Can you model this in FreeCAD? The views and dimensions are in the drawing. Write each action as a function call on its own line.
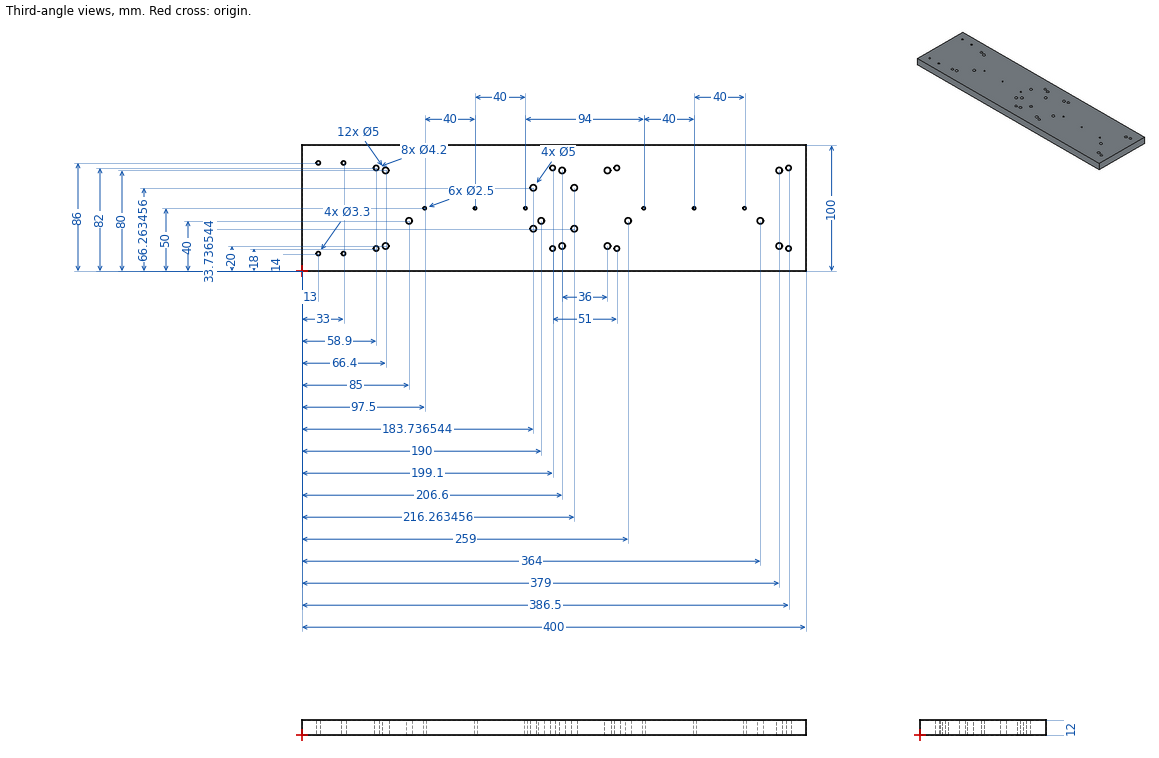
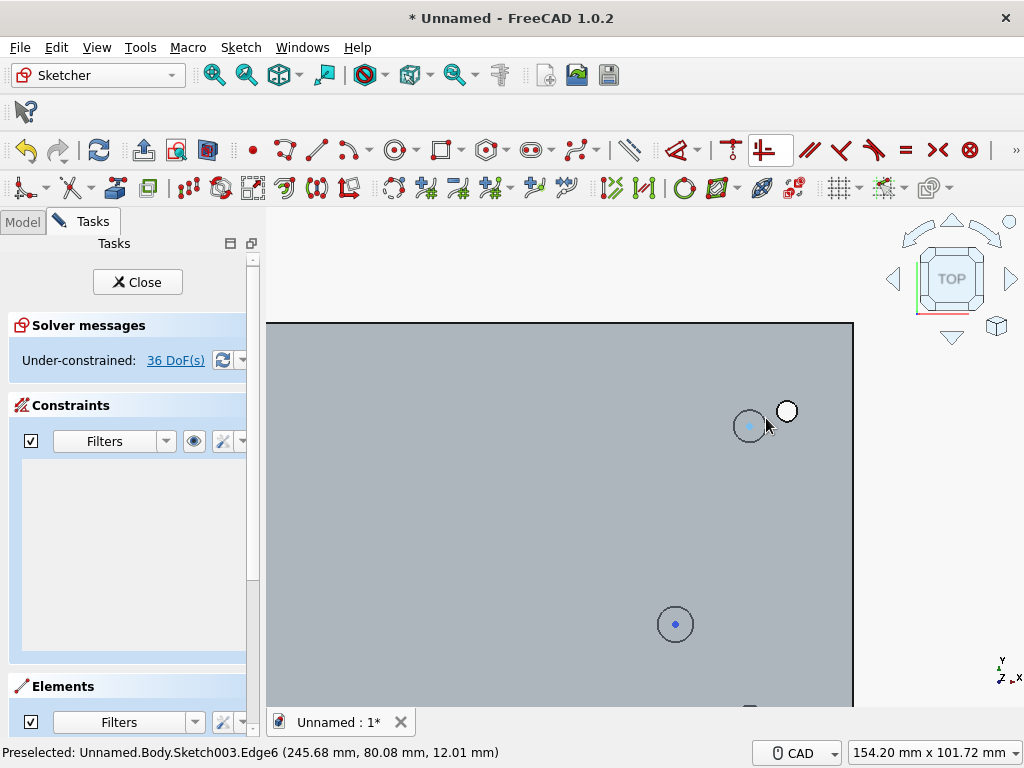
click(761, 415)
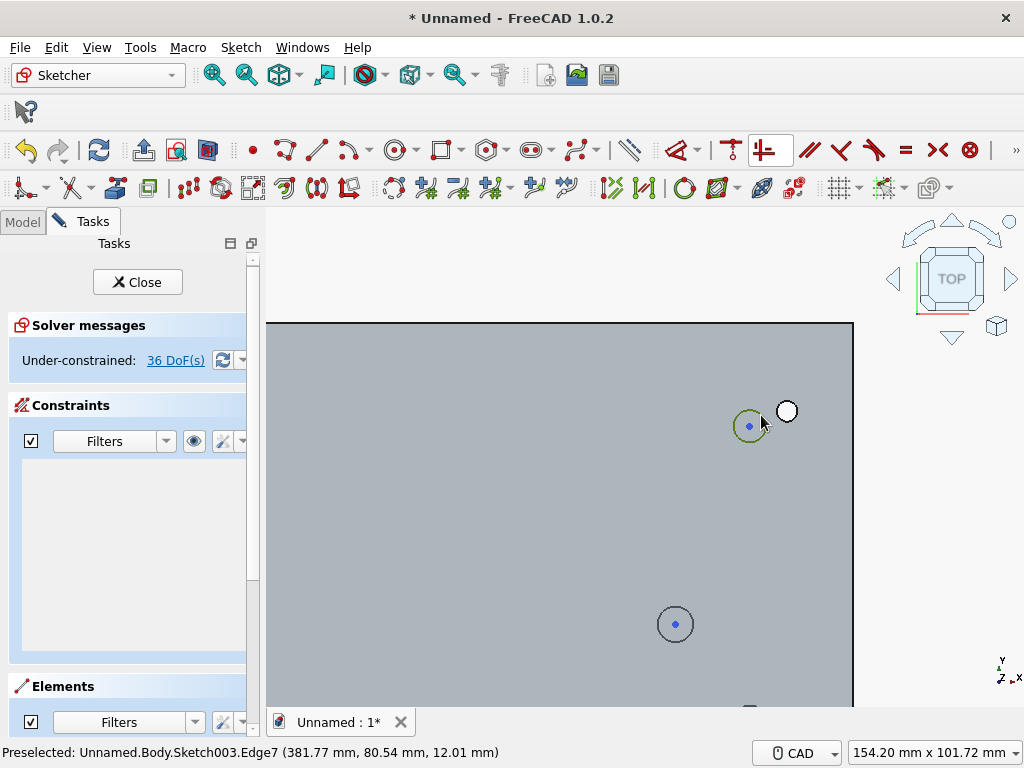
scroll(767, 418, down, 8)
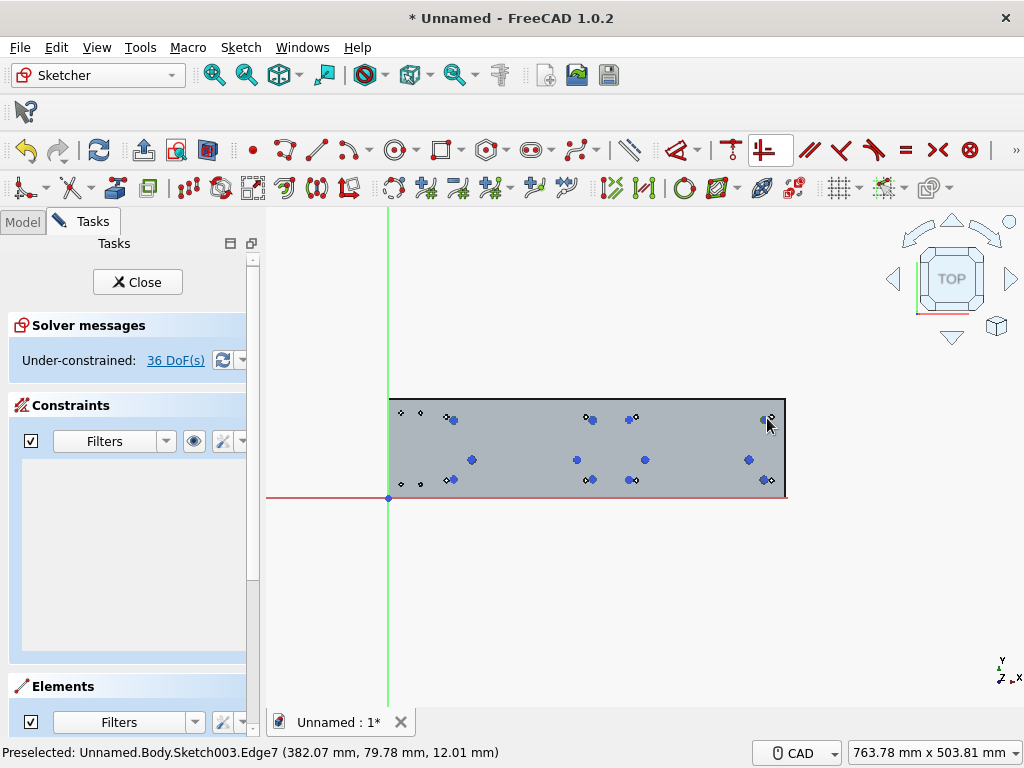
scroll(767, 477, up, 7)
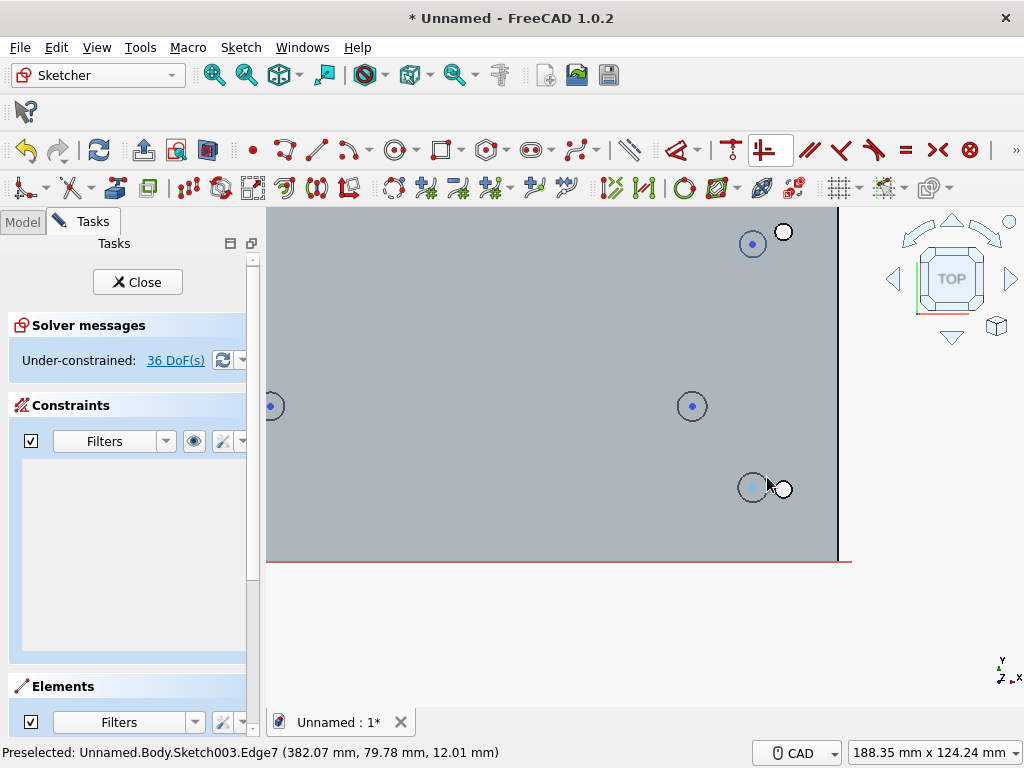
click(763, 477)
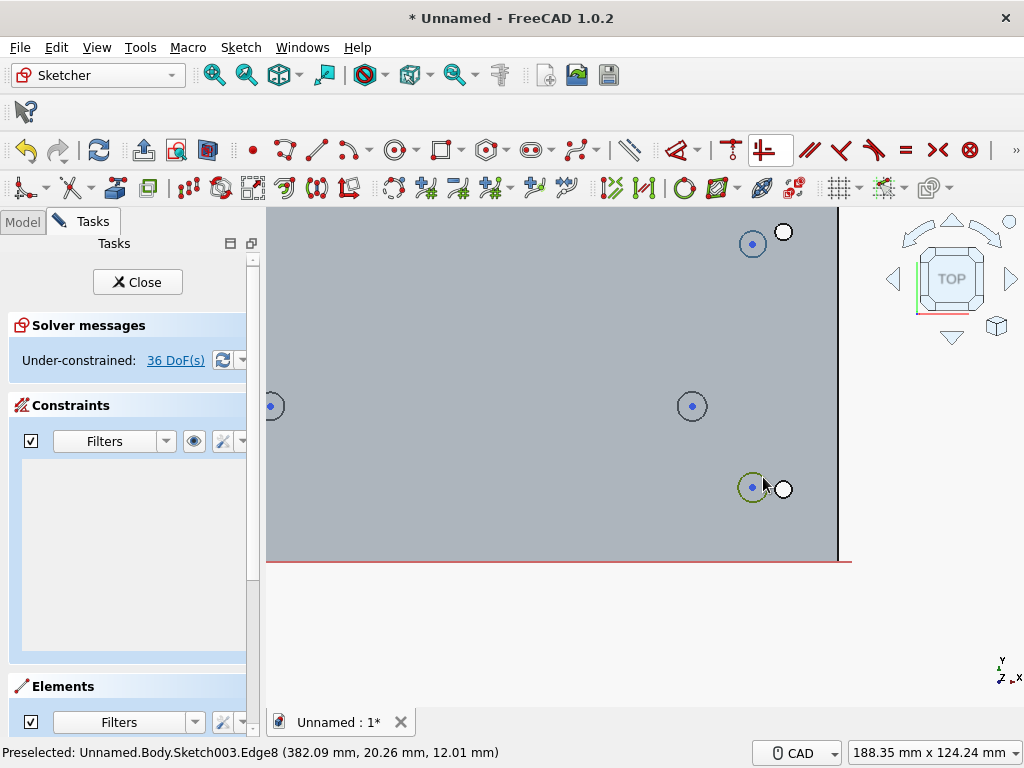
scroll(767, 477, down, 7)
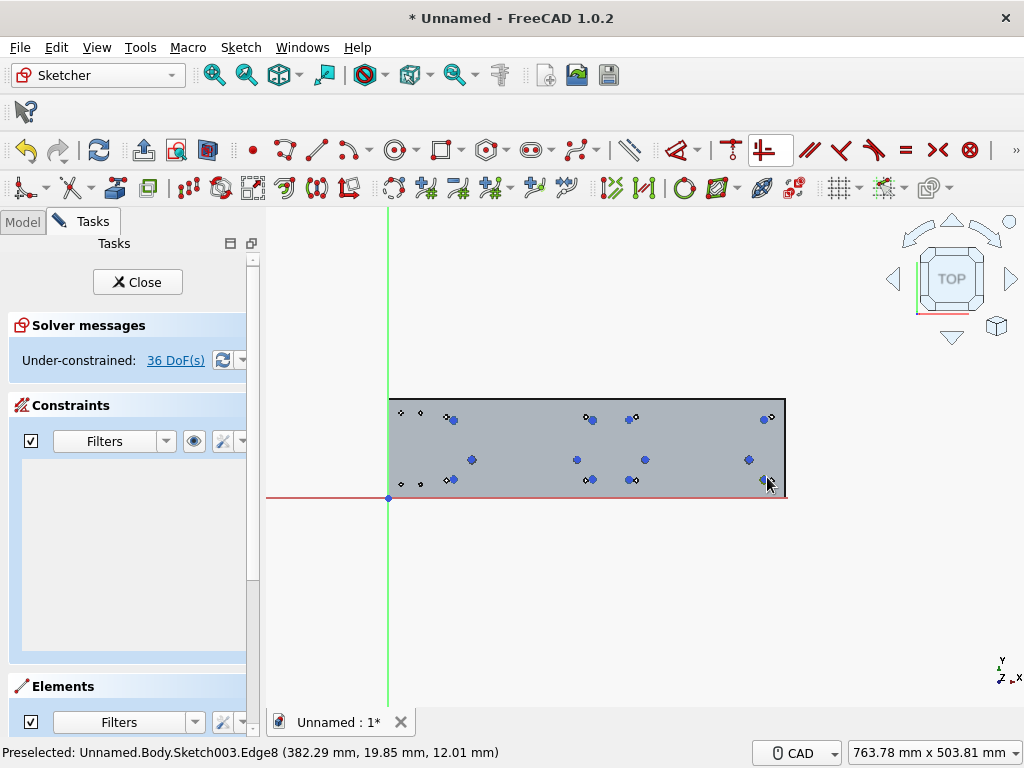
scroll(475, 457, up, 7)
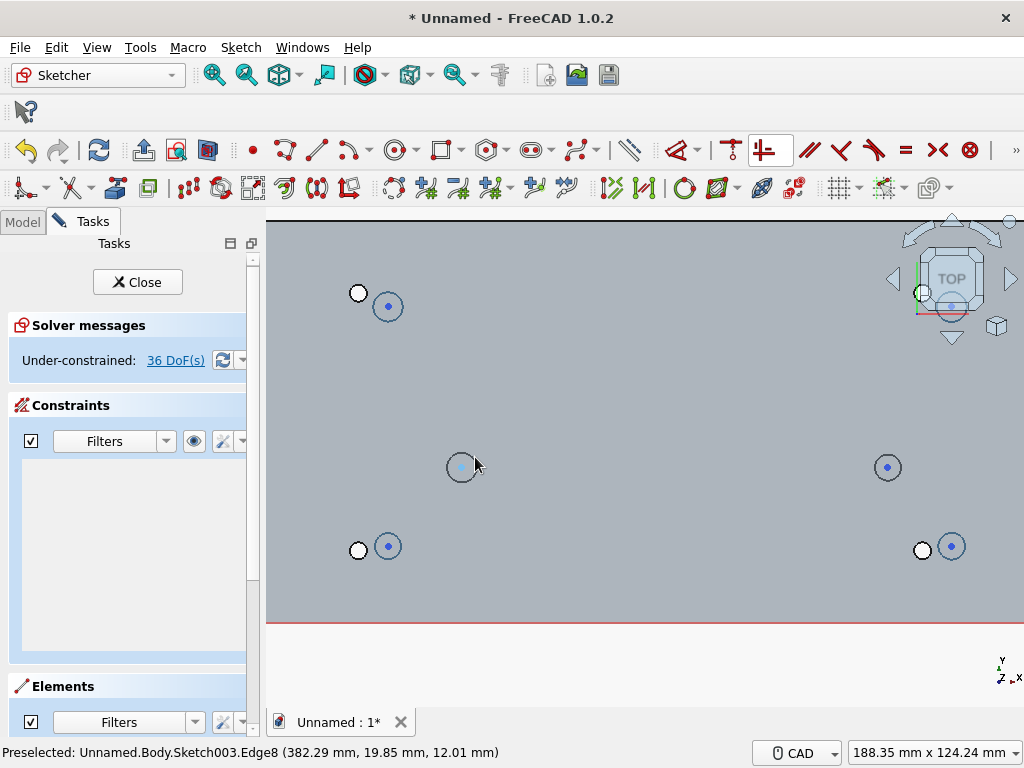
click(472, 457)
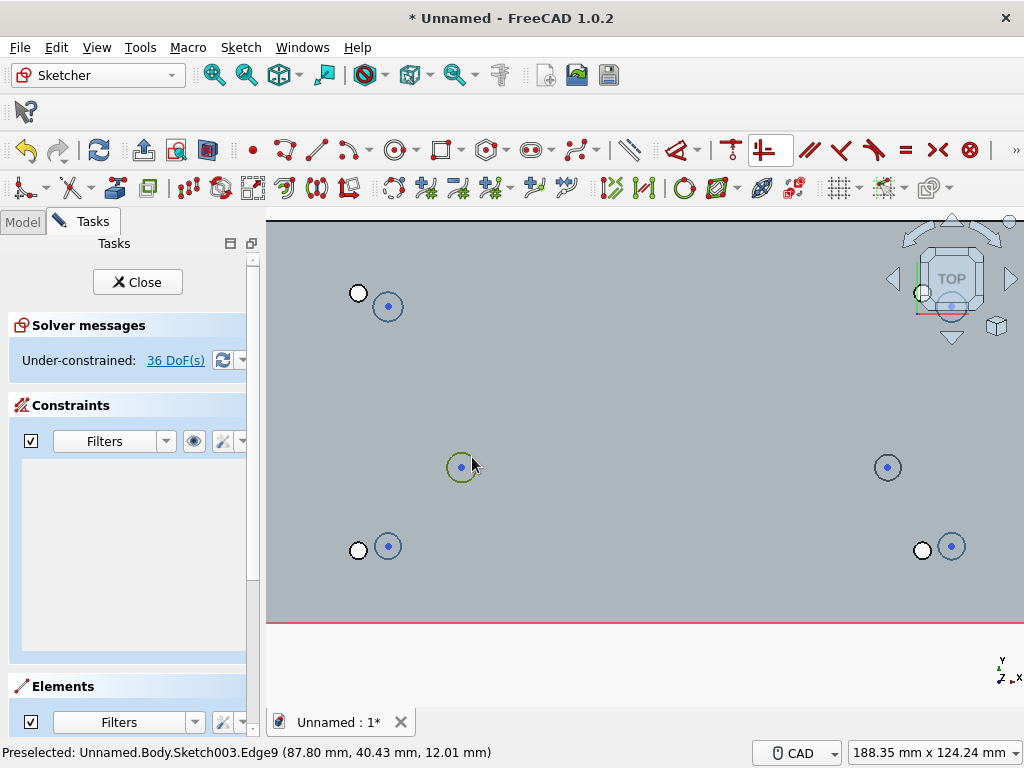
scroll(474, 457, down, 7)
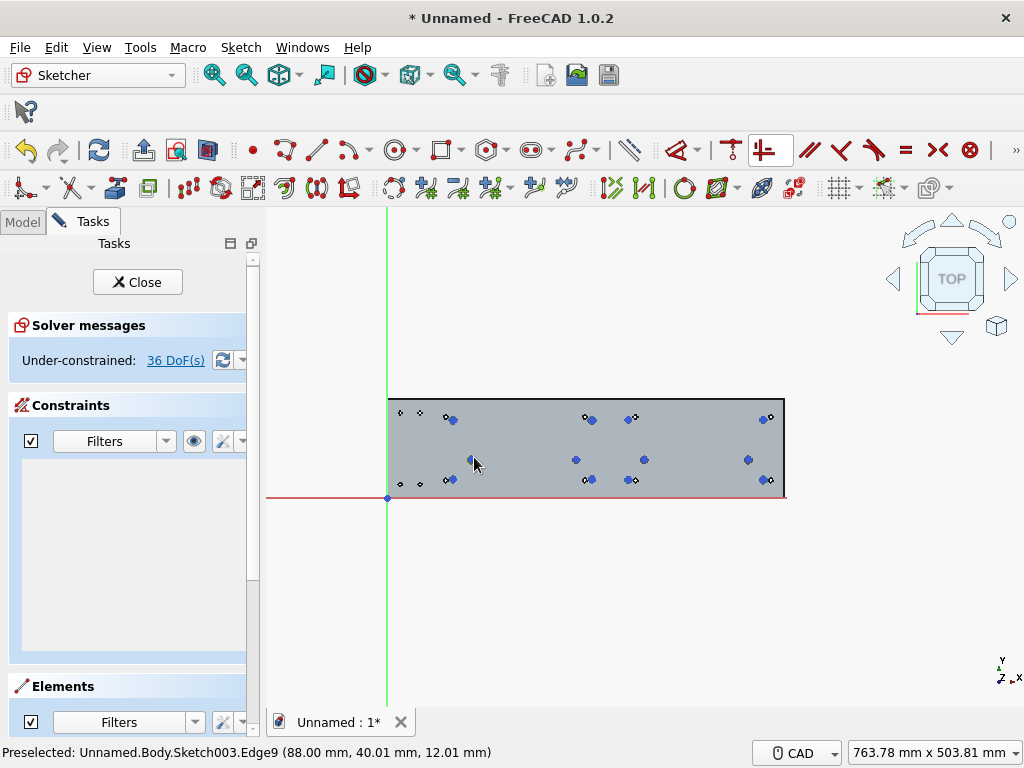
scroll(579, 458, up, 8)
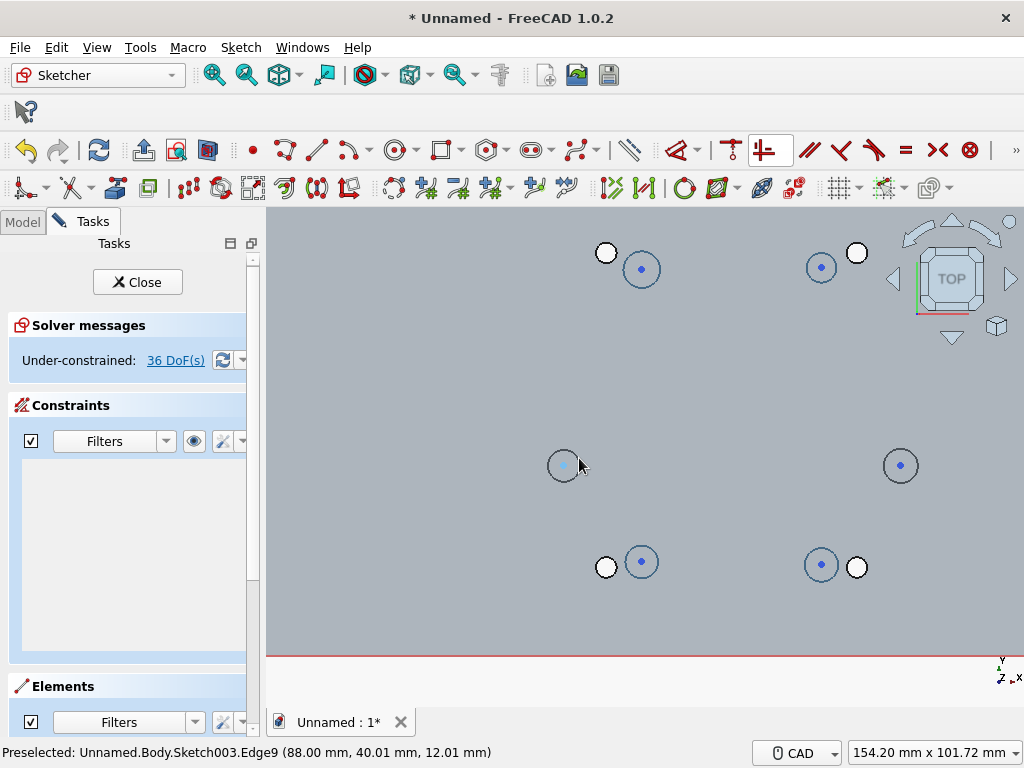
click(575, 455)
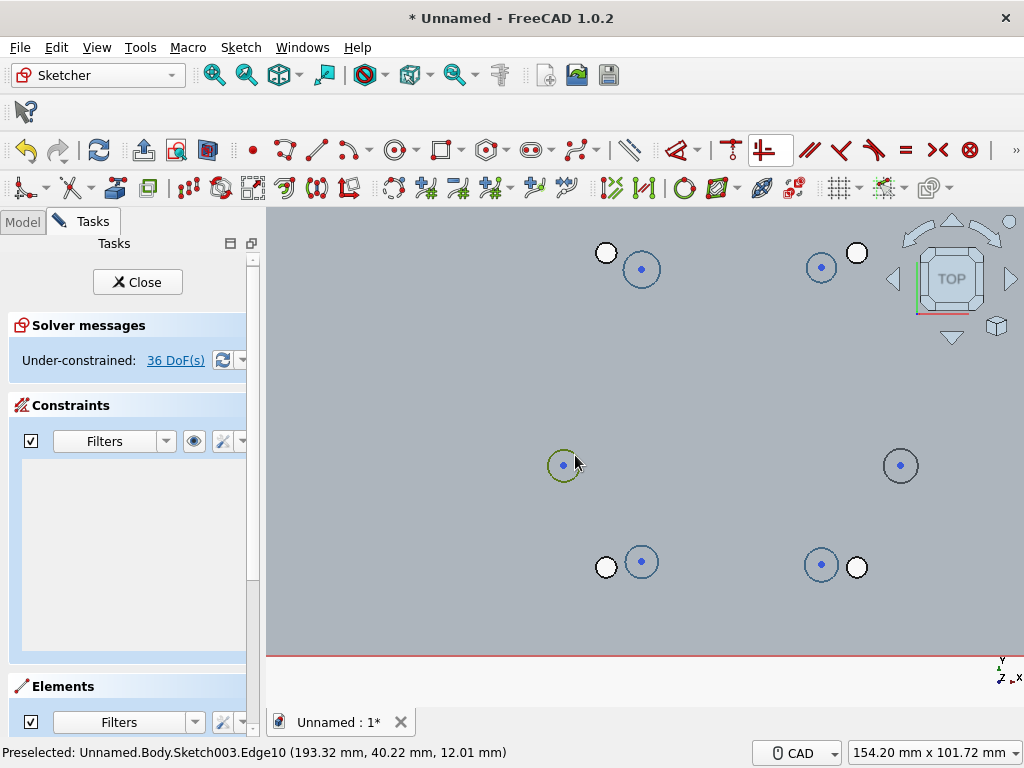
scroll(579, 458, down, 8)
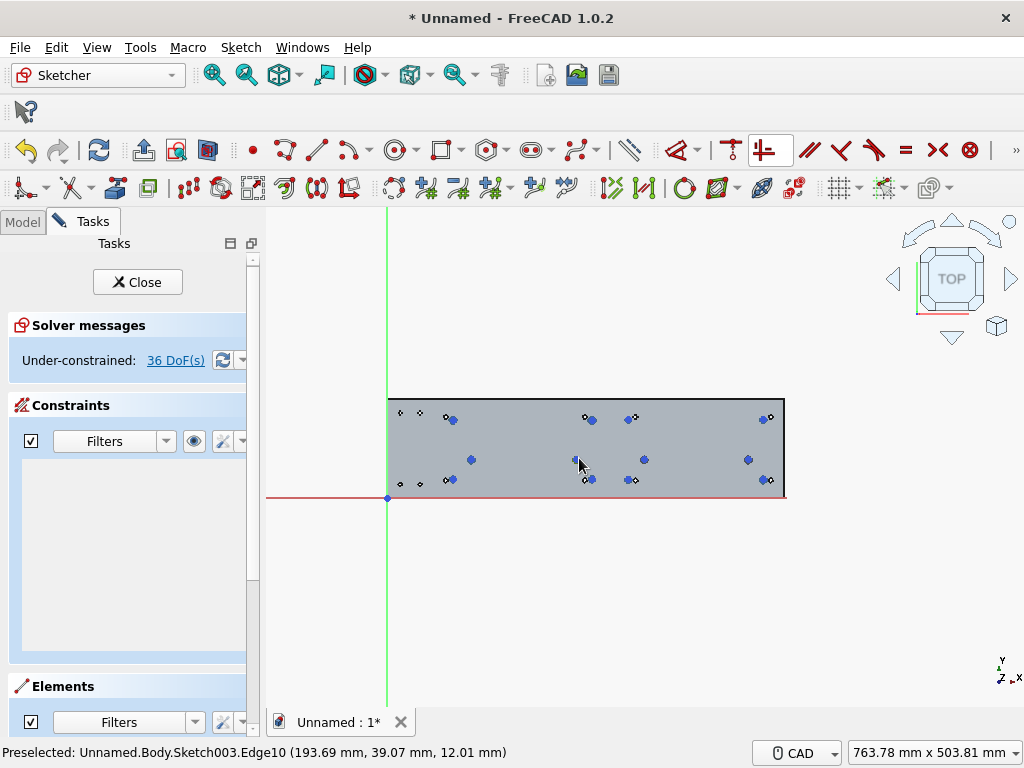
scroll(647, 458, up, 7)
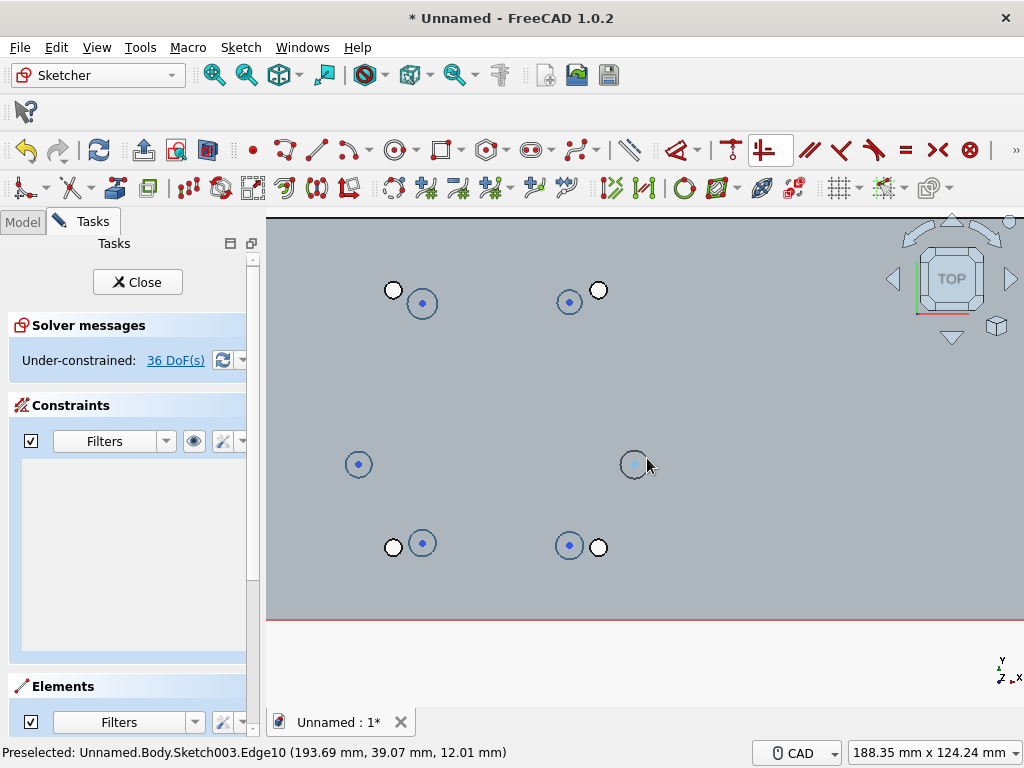
click(644, 455)